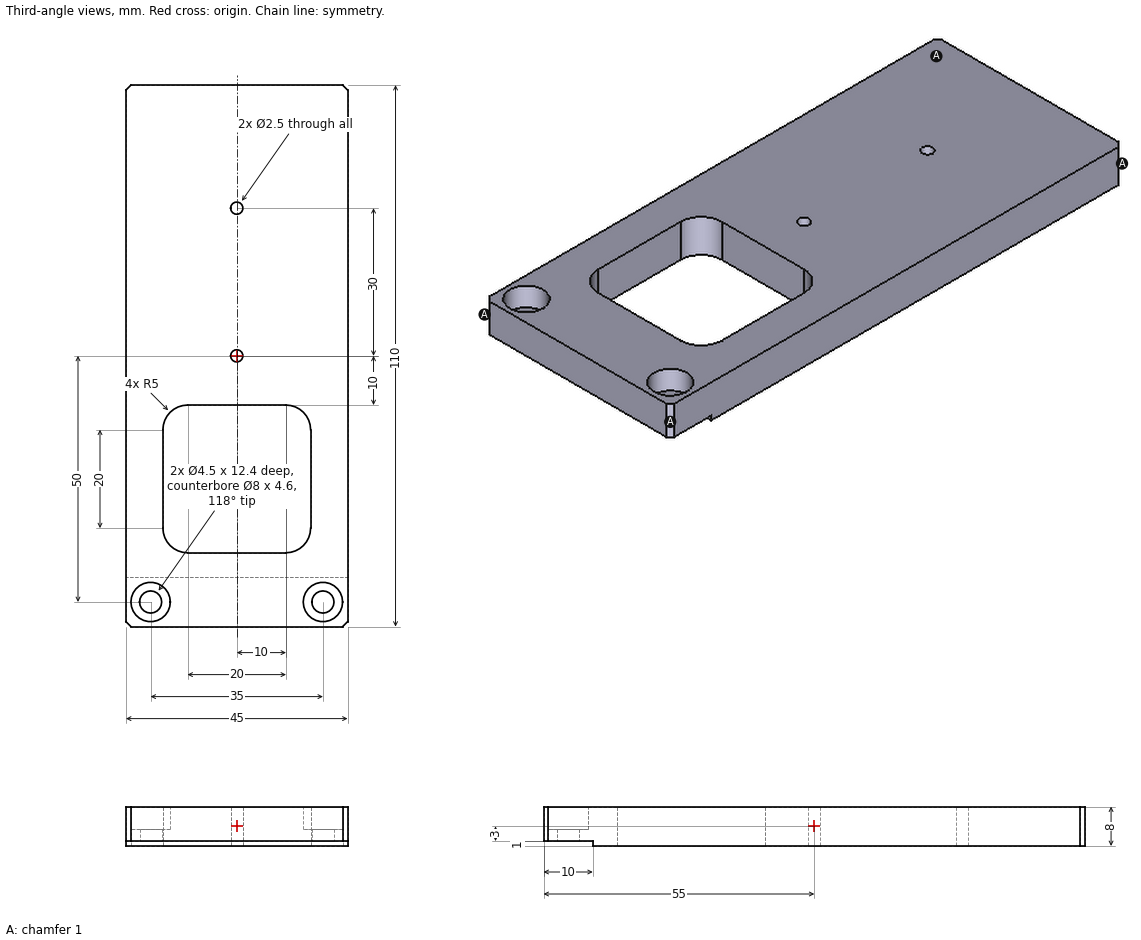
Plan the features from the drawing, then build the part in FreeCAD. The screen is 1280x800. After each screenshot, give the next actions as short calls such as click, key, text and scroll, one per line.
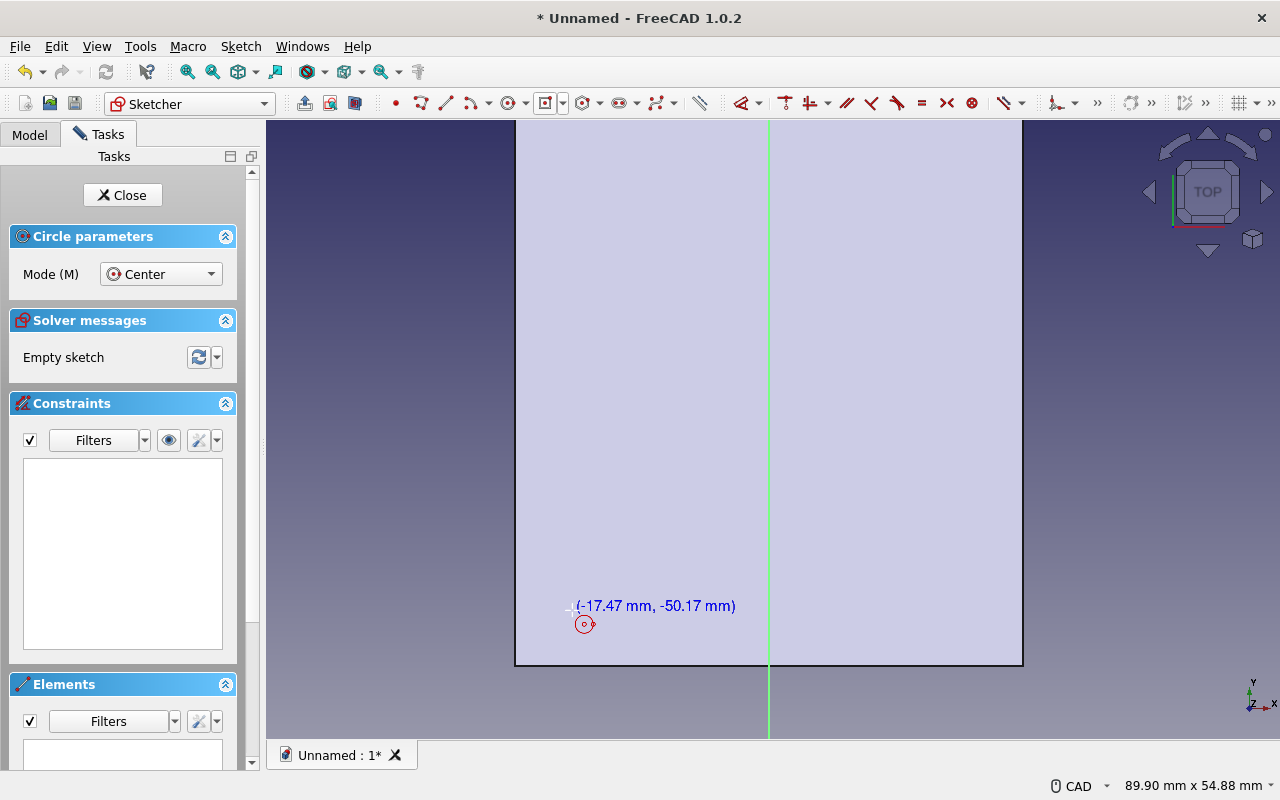
click(571, 609)
move(589, 591)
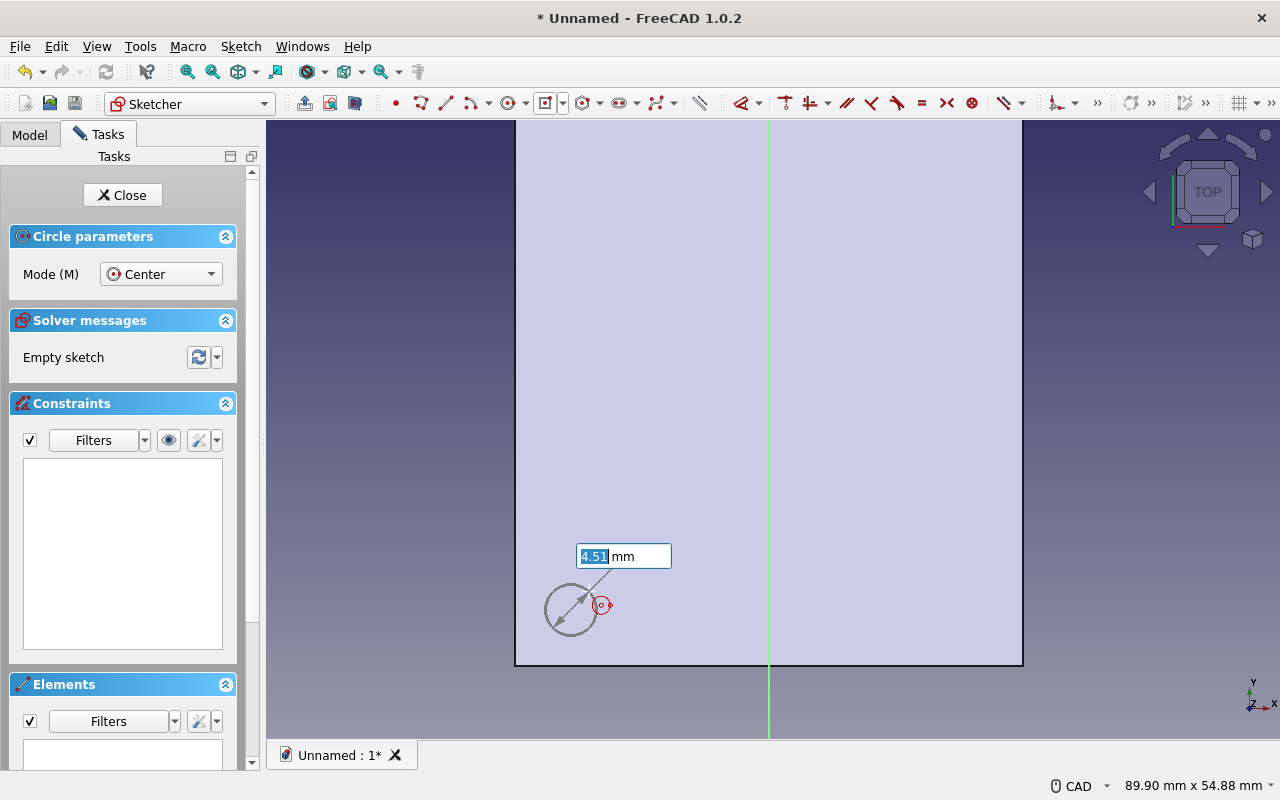
text(4.5)
key(Return)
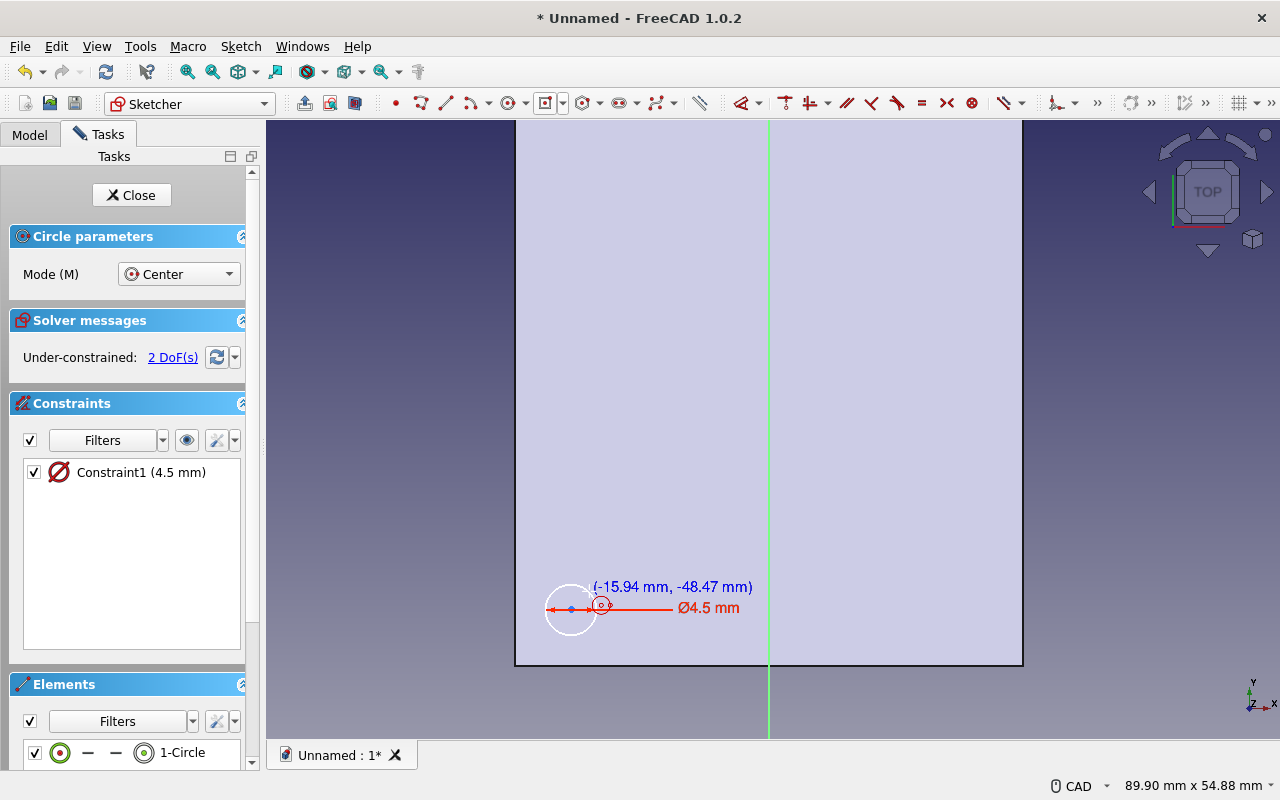
click(966, 609)
move(984, 591)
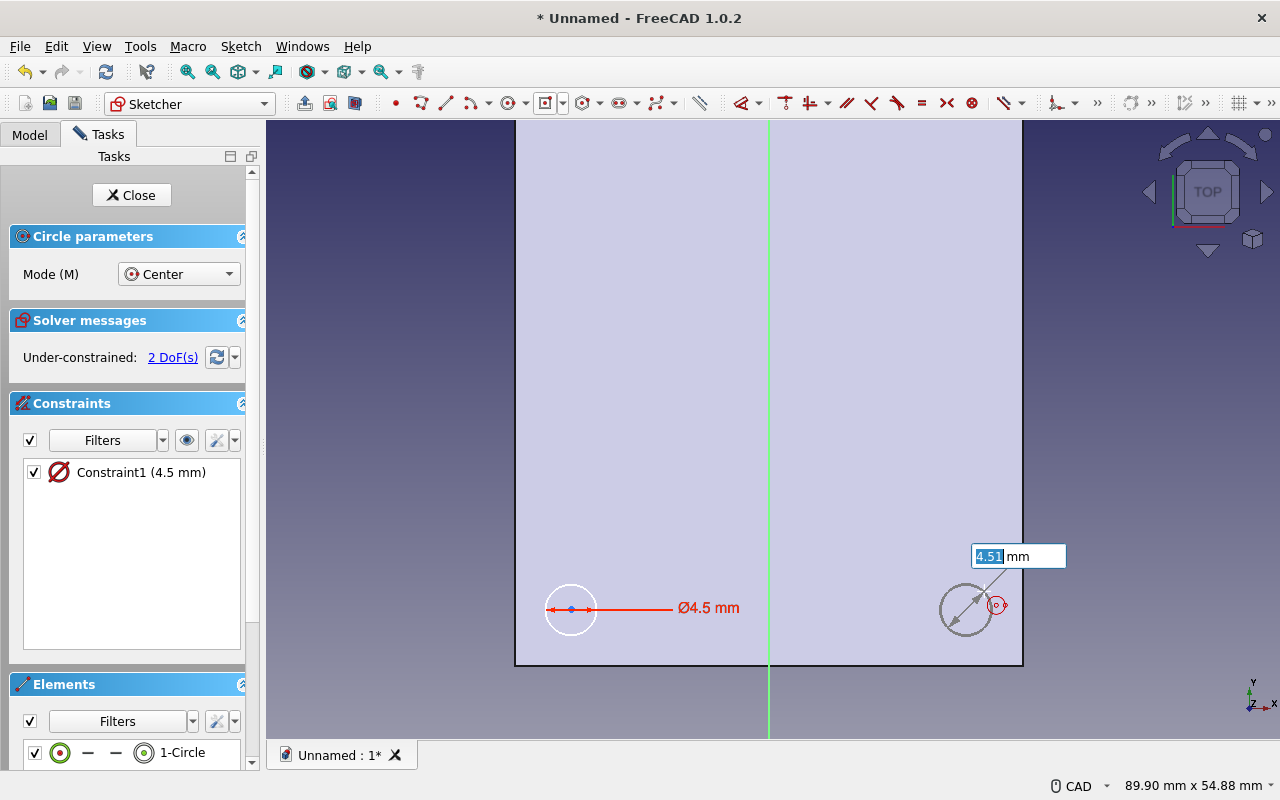
text(4.5)
key(Return)
key(Escape)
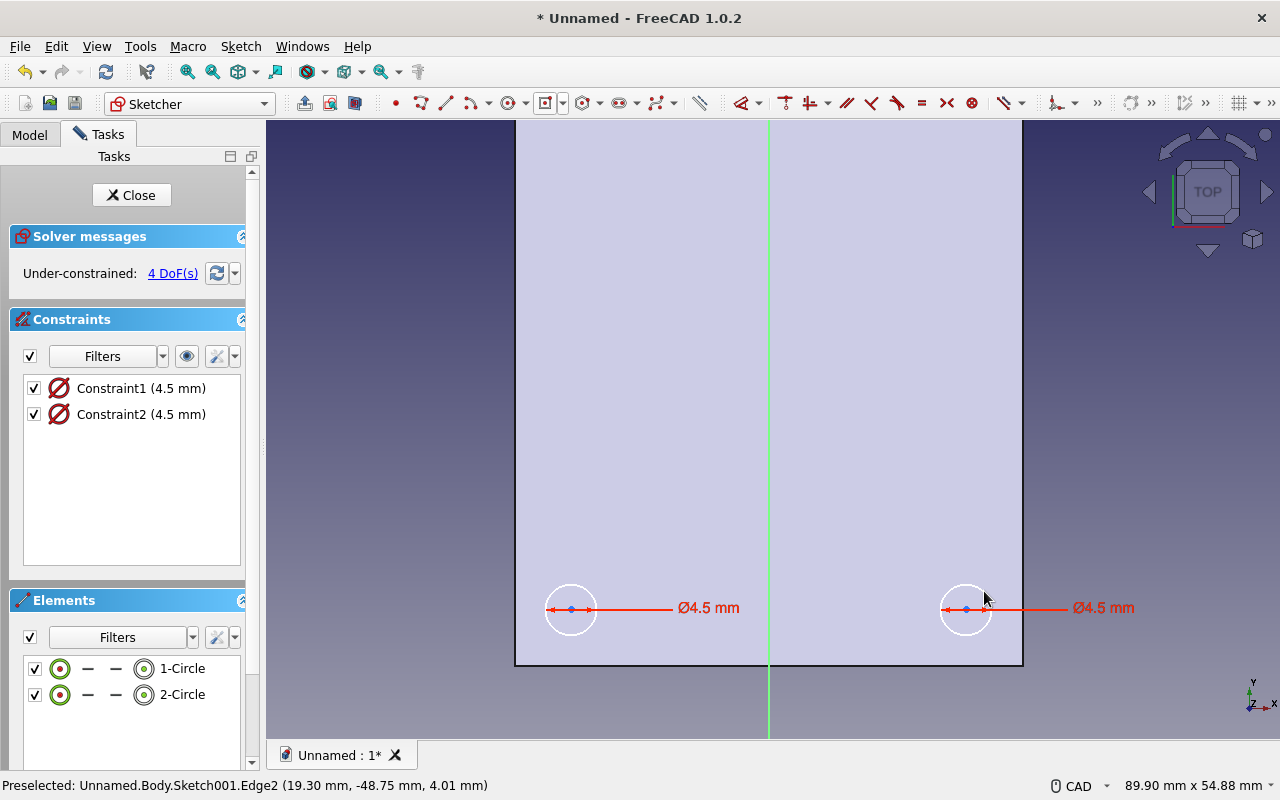
click(571, 610)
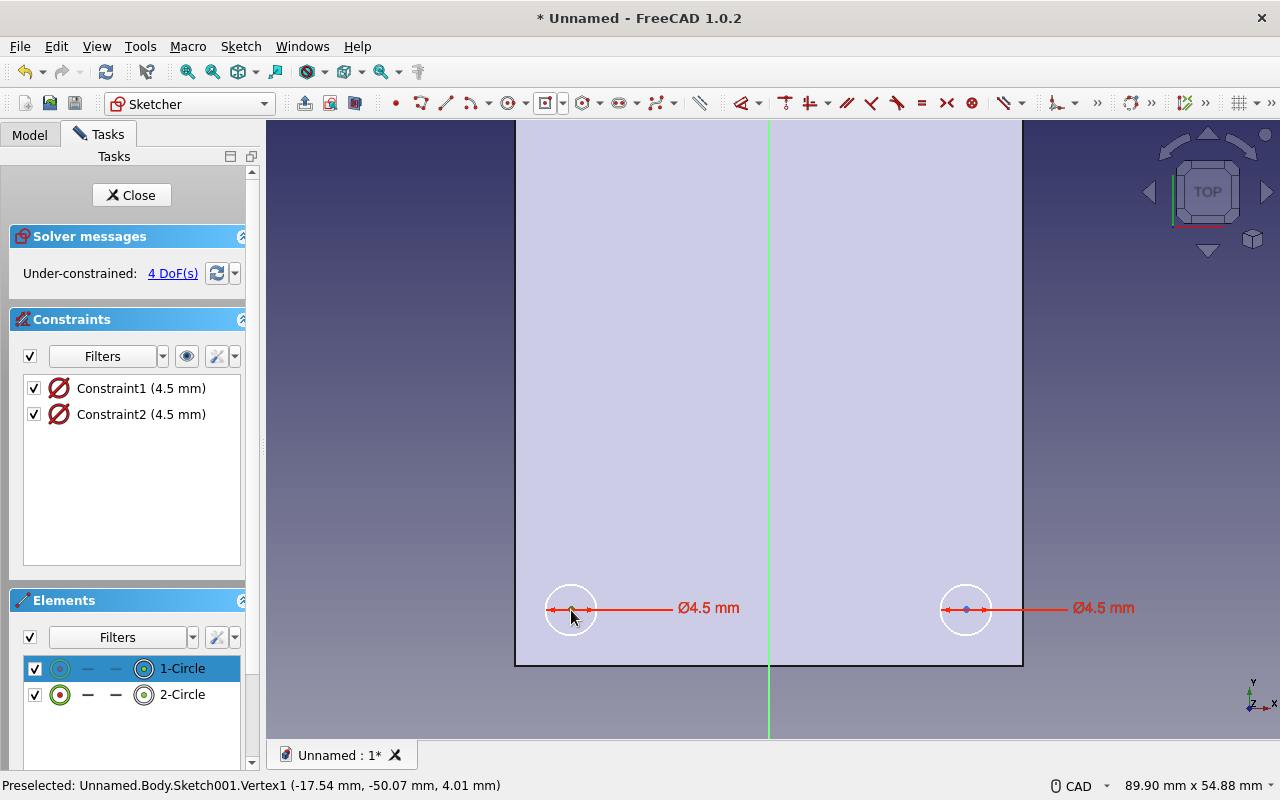
click(966, 610)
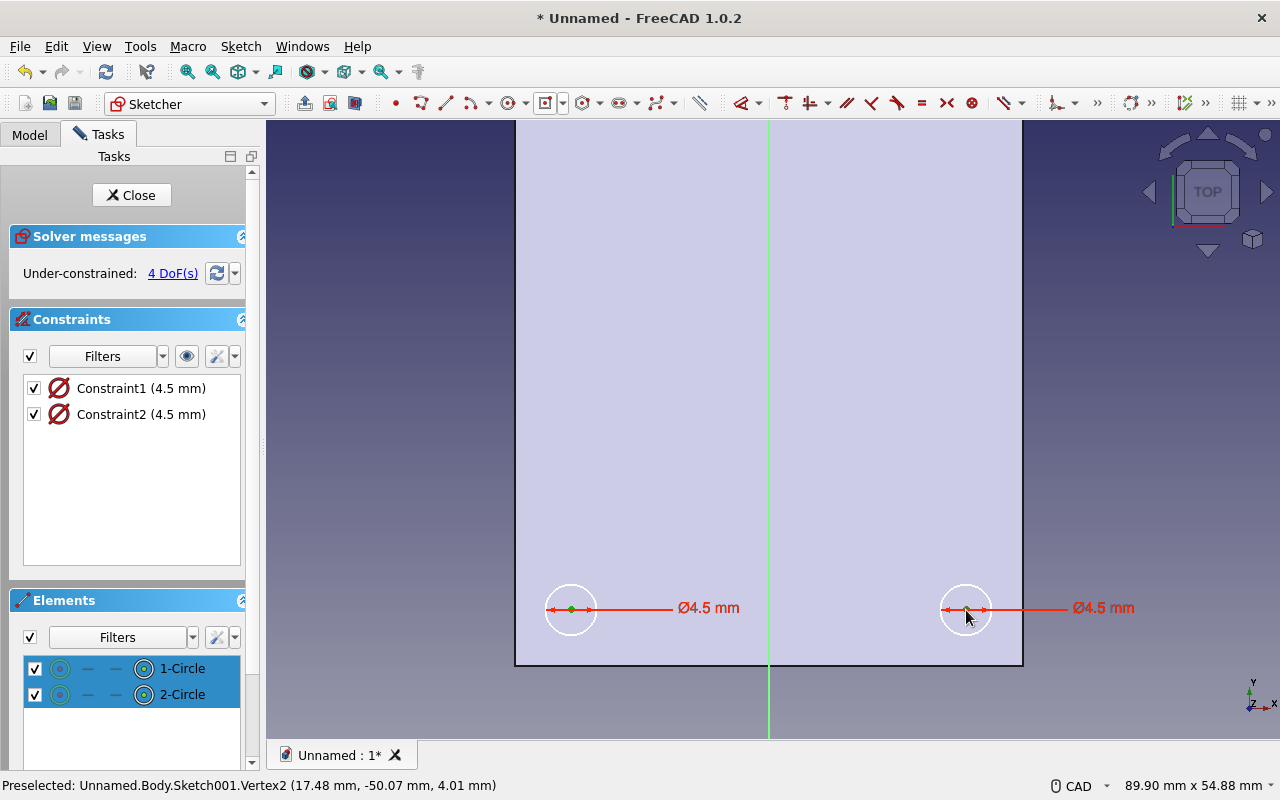
click(769, 671)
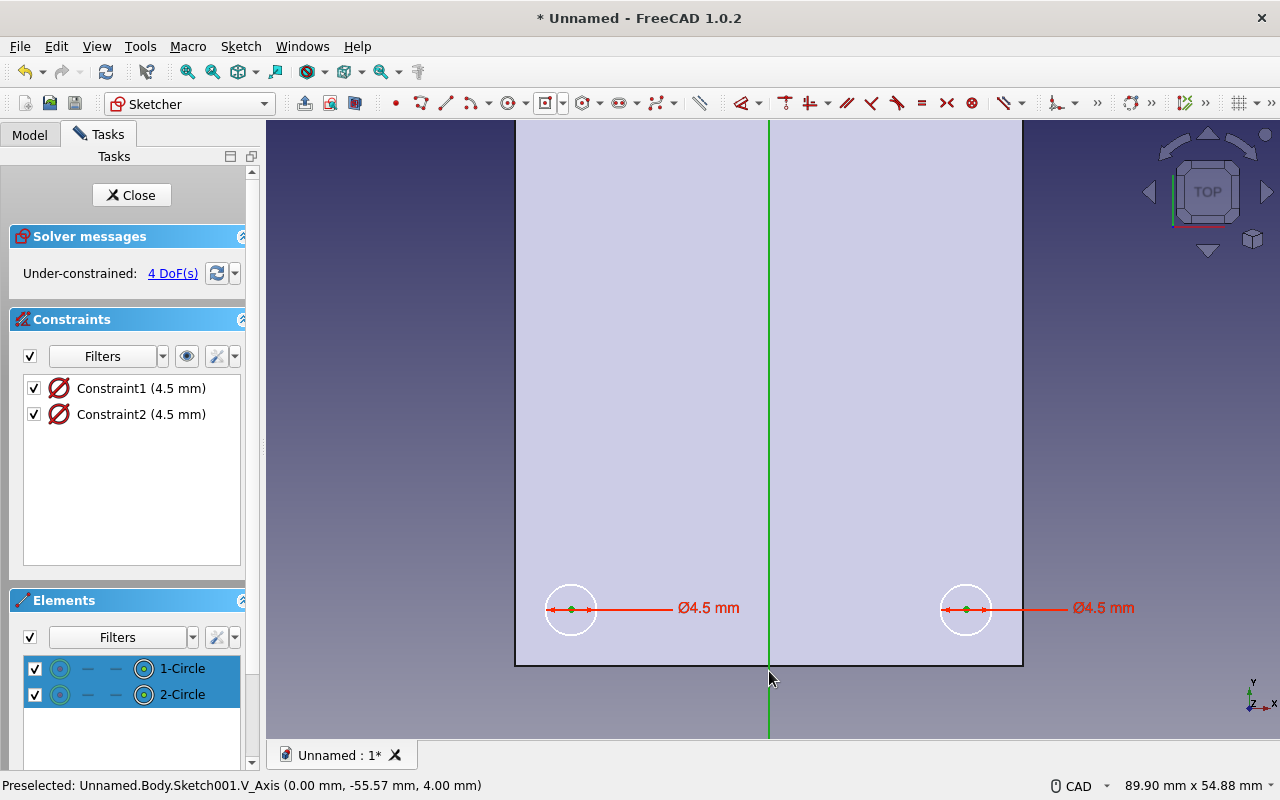
click(947, 104)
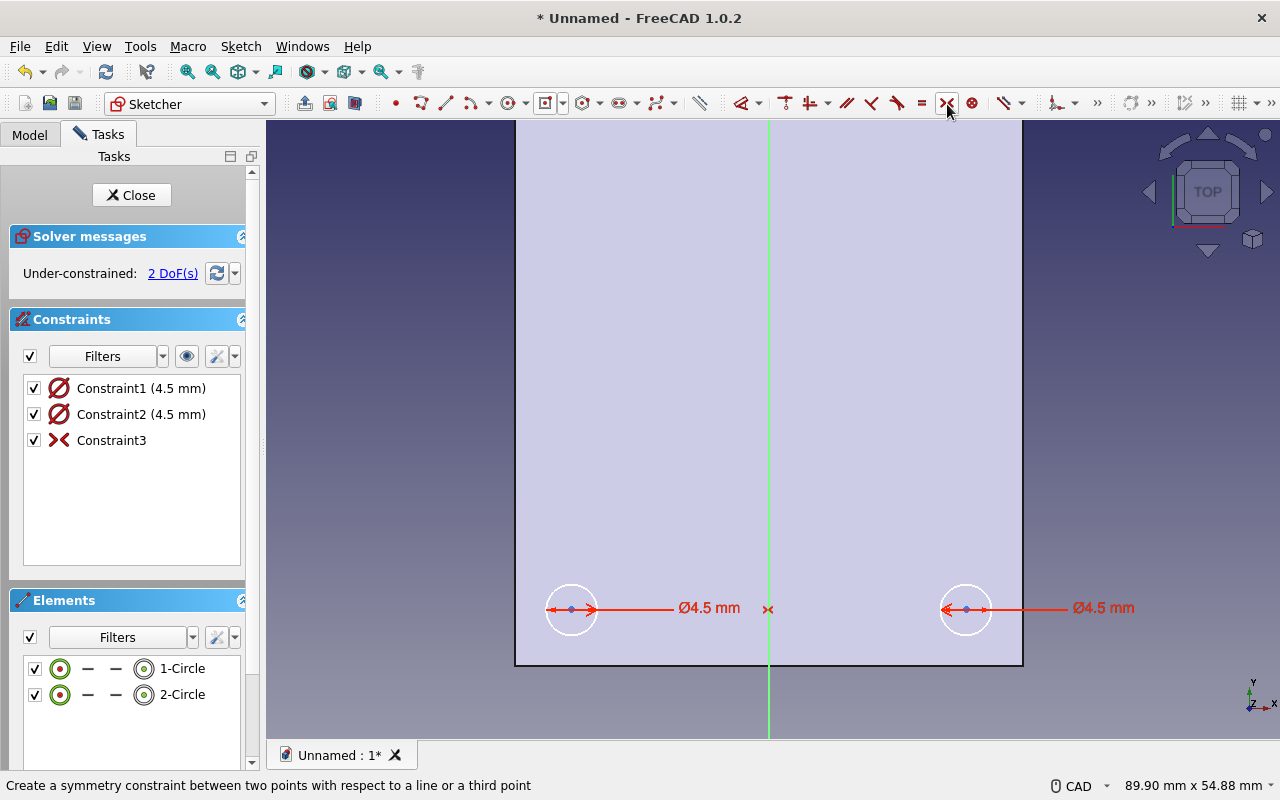
click(572, 610)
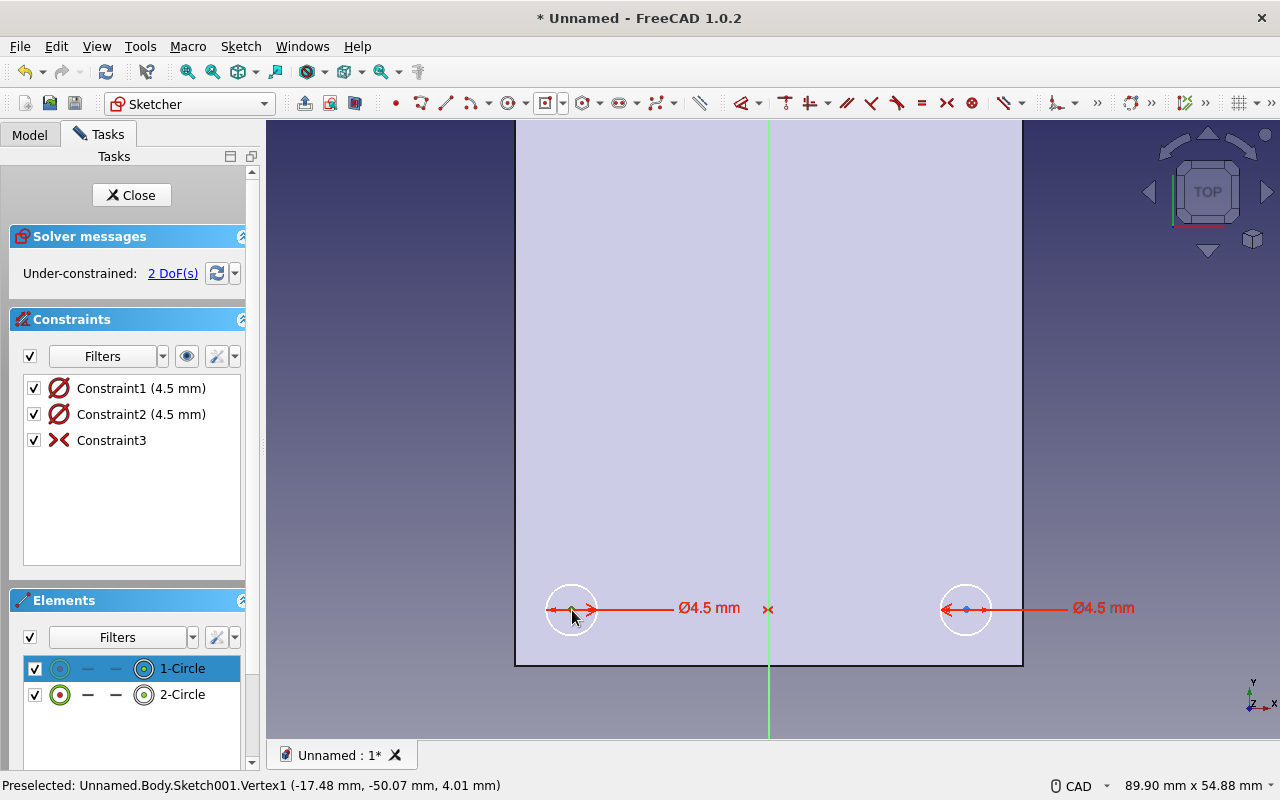
click(758, 104)